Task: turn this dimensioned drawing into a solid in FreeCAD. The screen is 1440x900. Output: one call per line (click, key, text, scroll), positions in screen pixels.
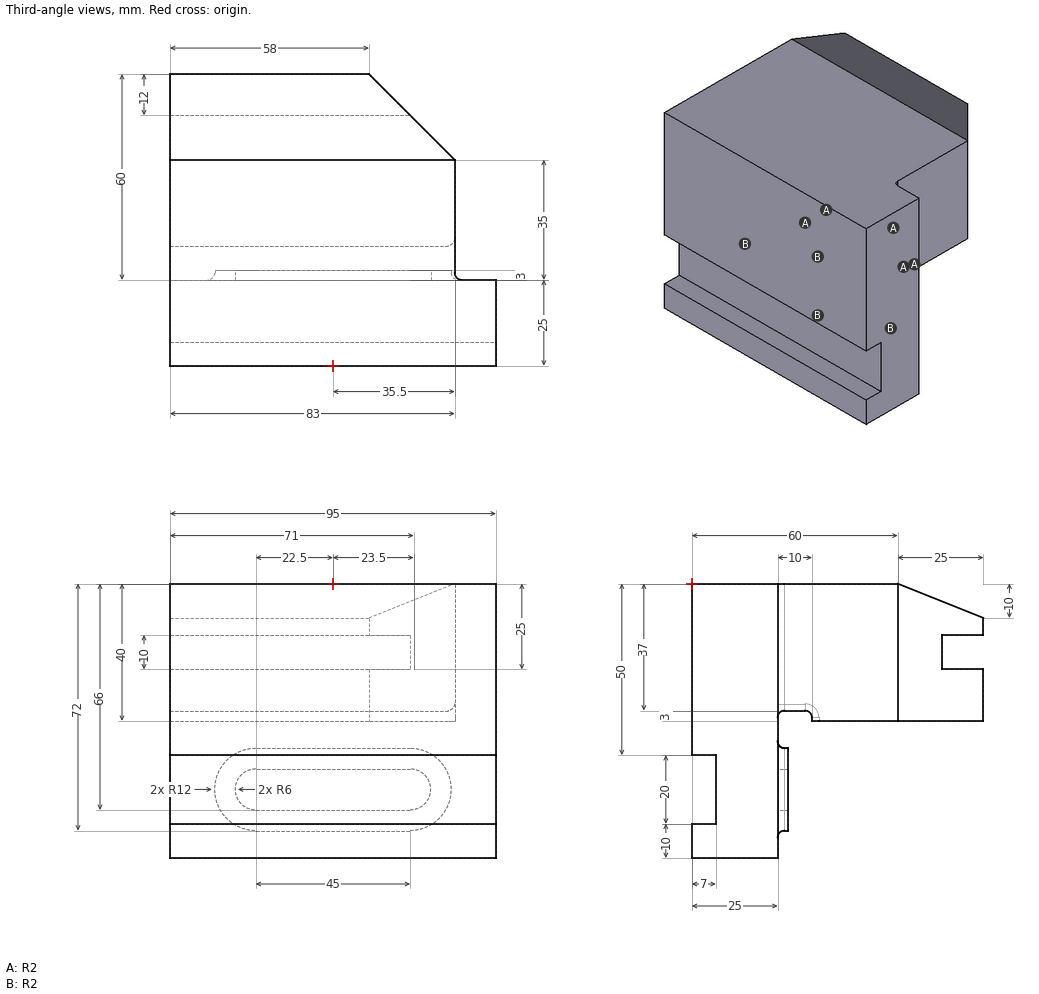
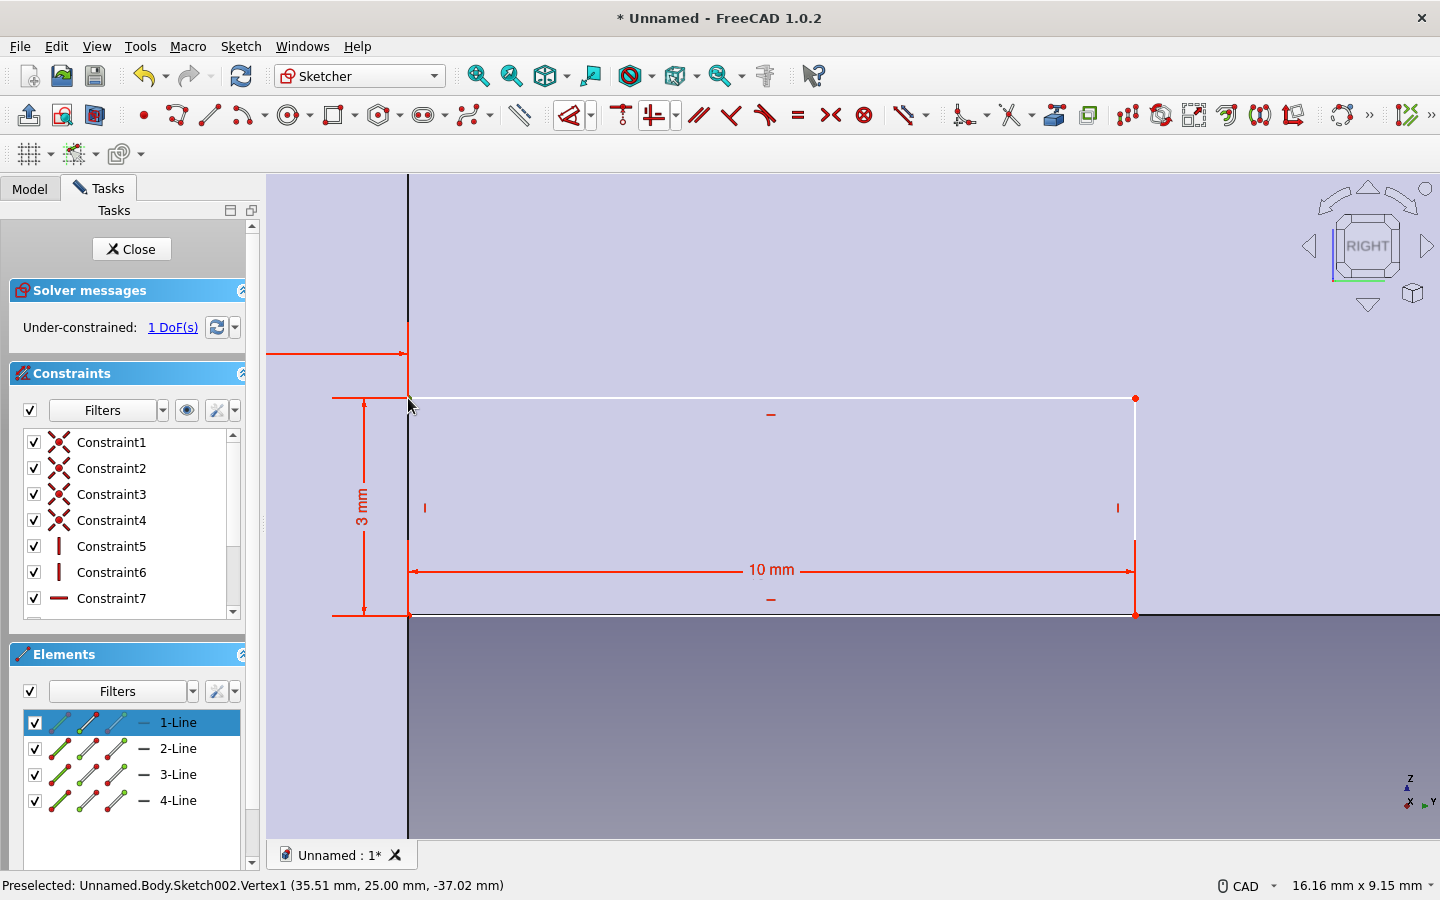
click(590, 116)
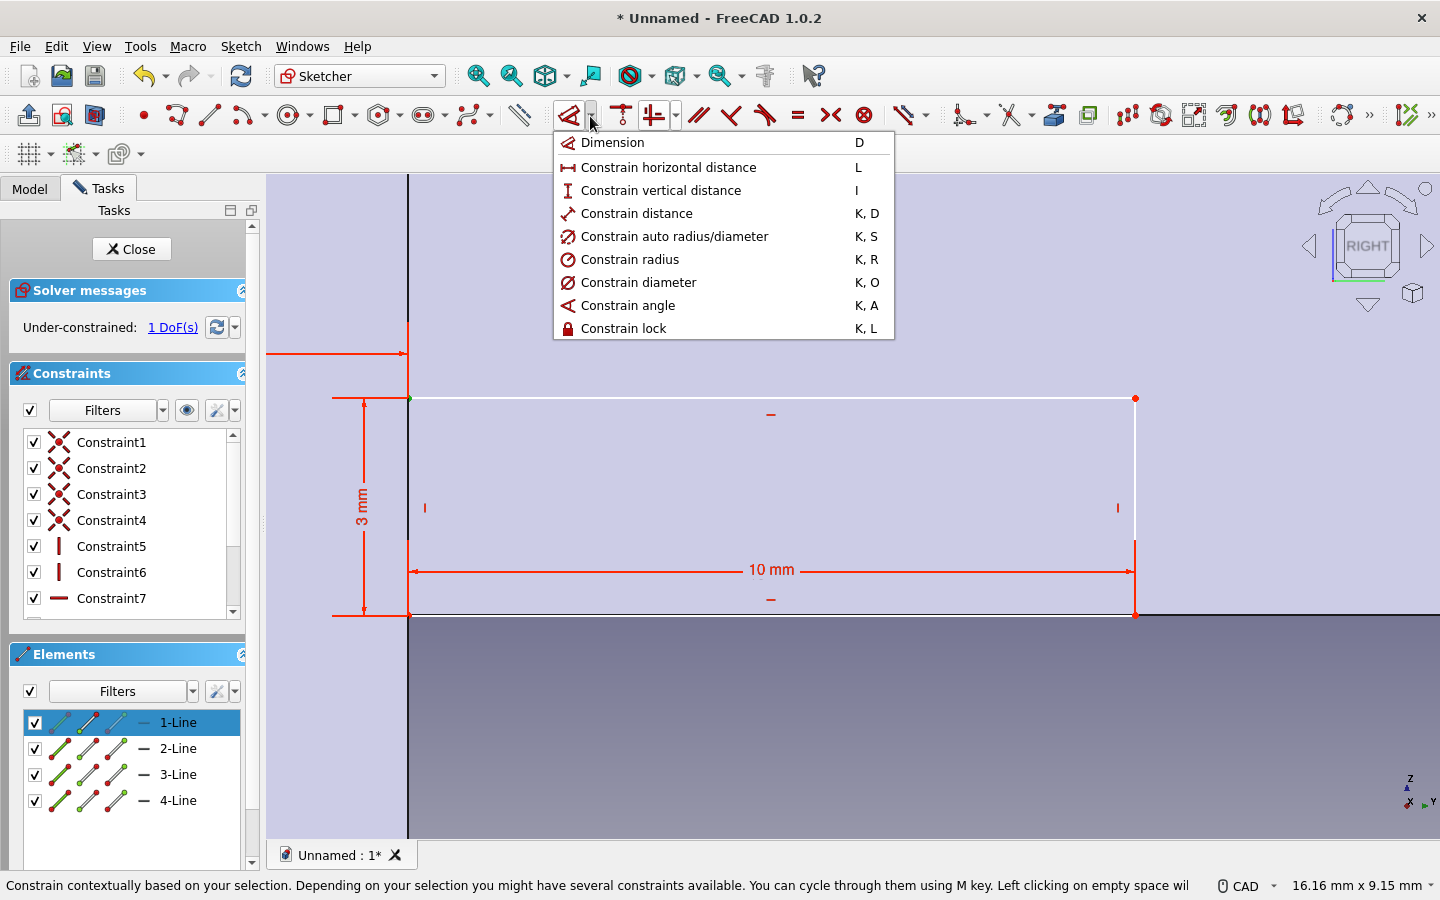
click(724, 190)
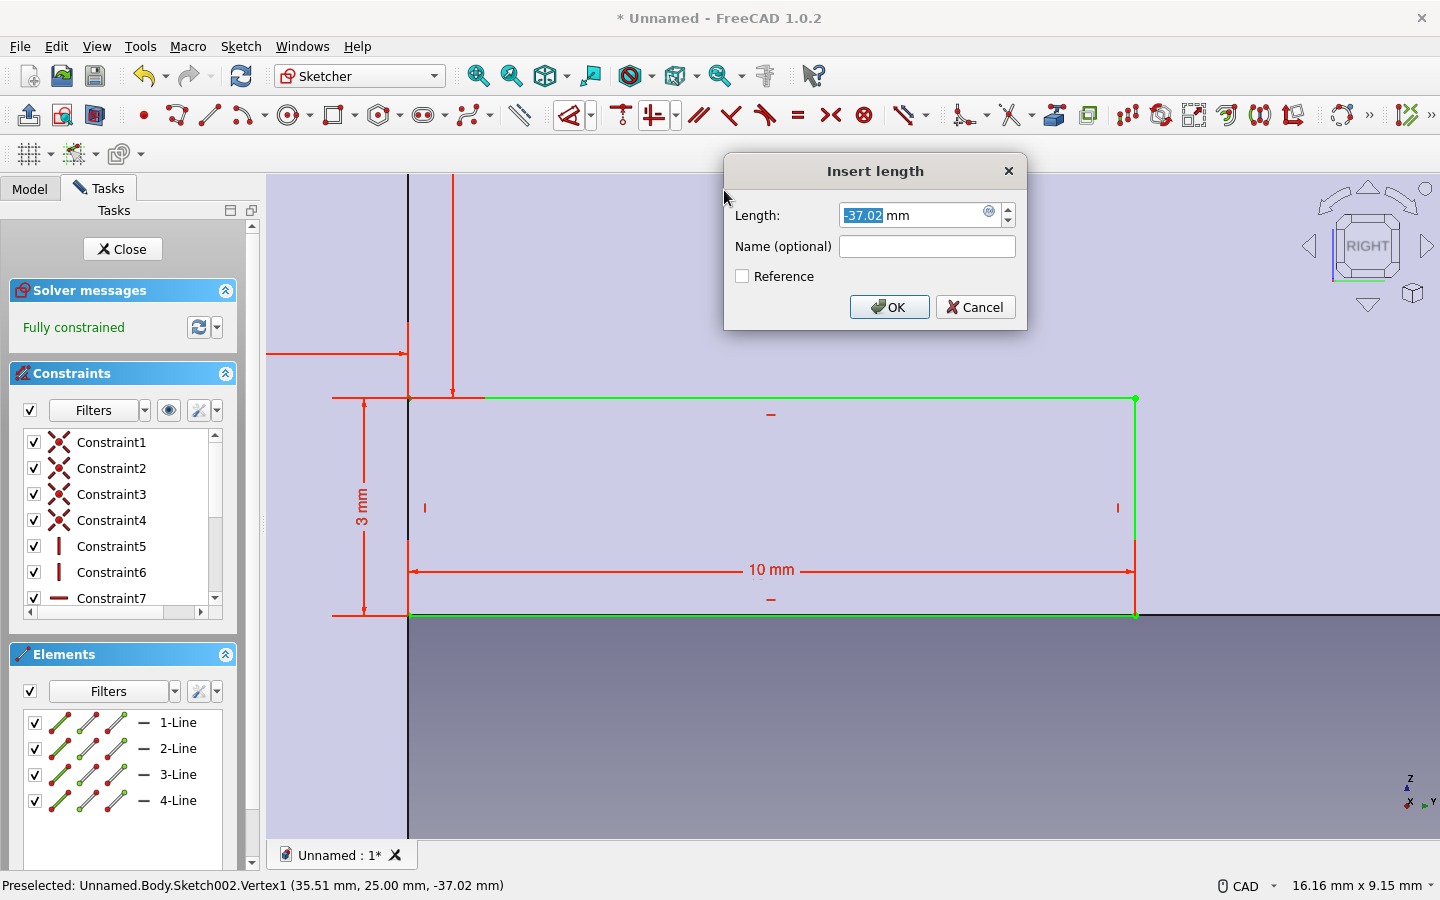
text(-37)
key(Return)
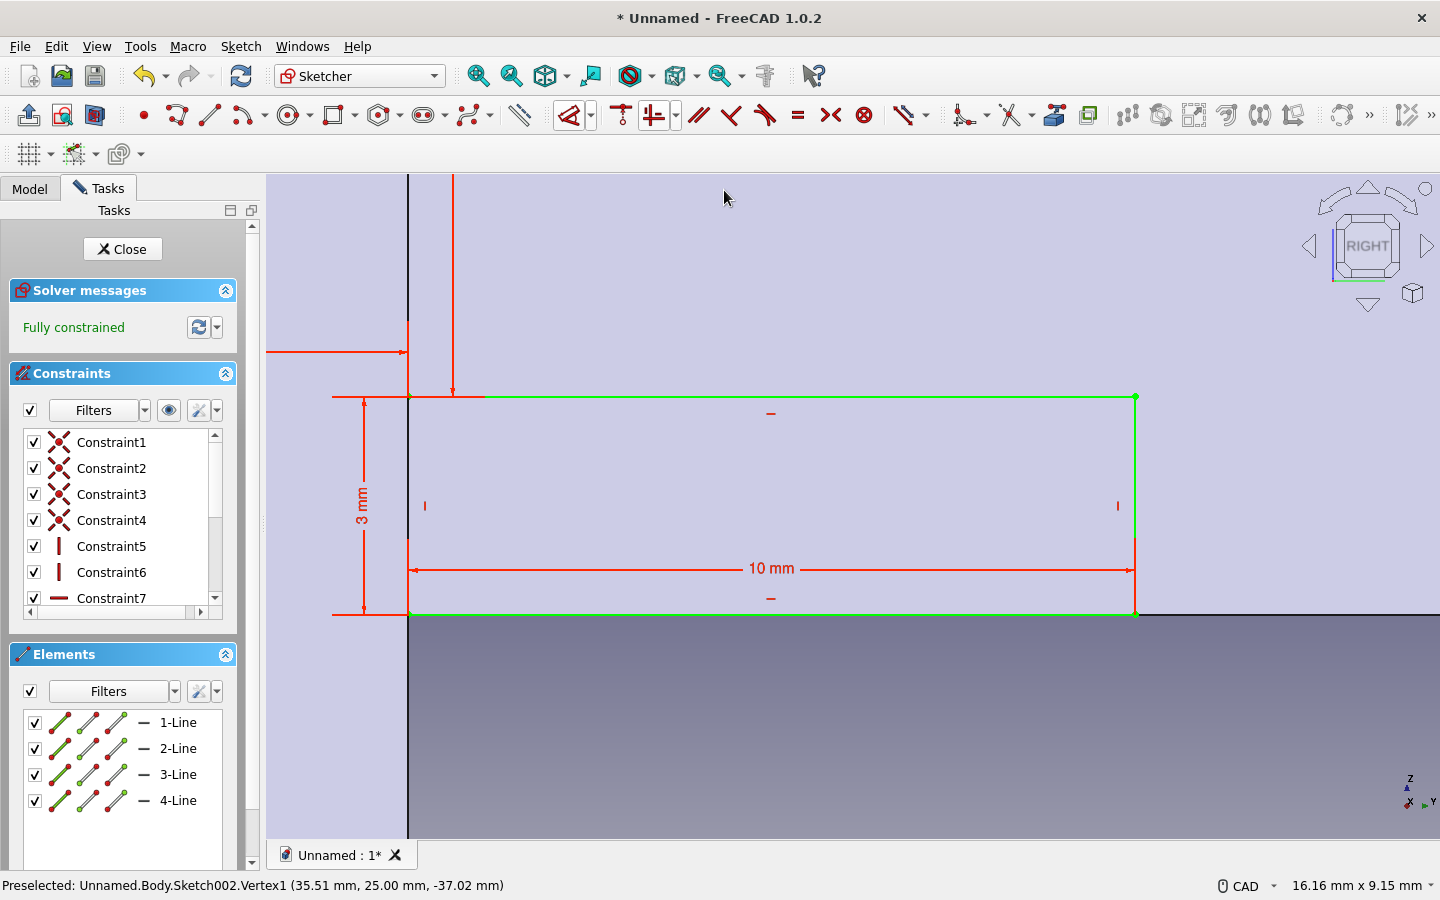
click(123, 249)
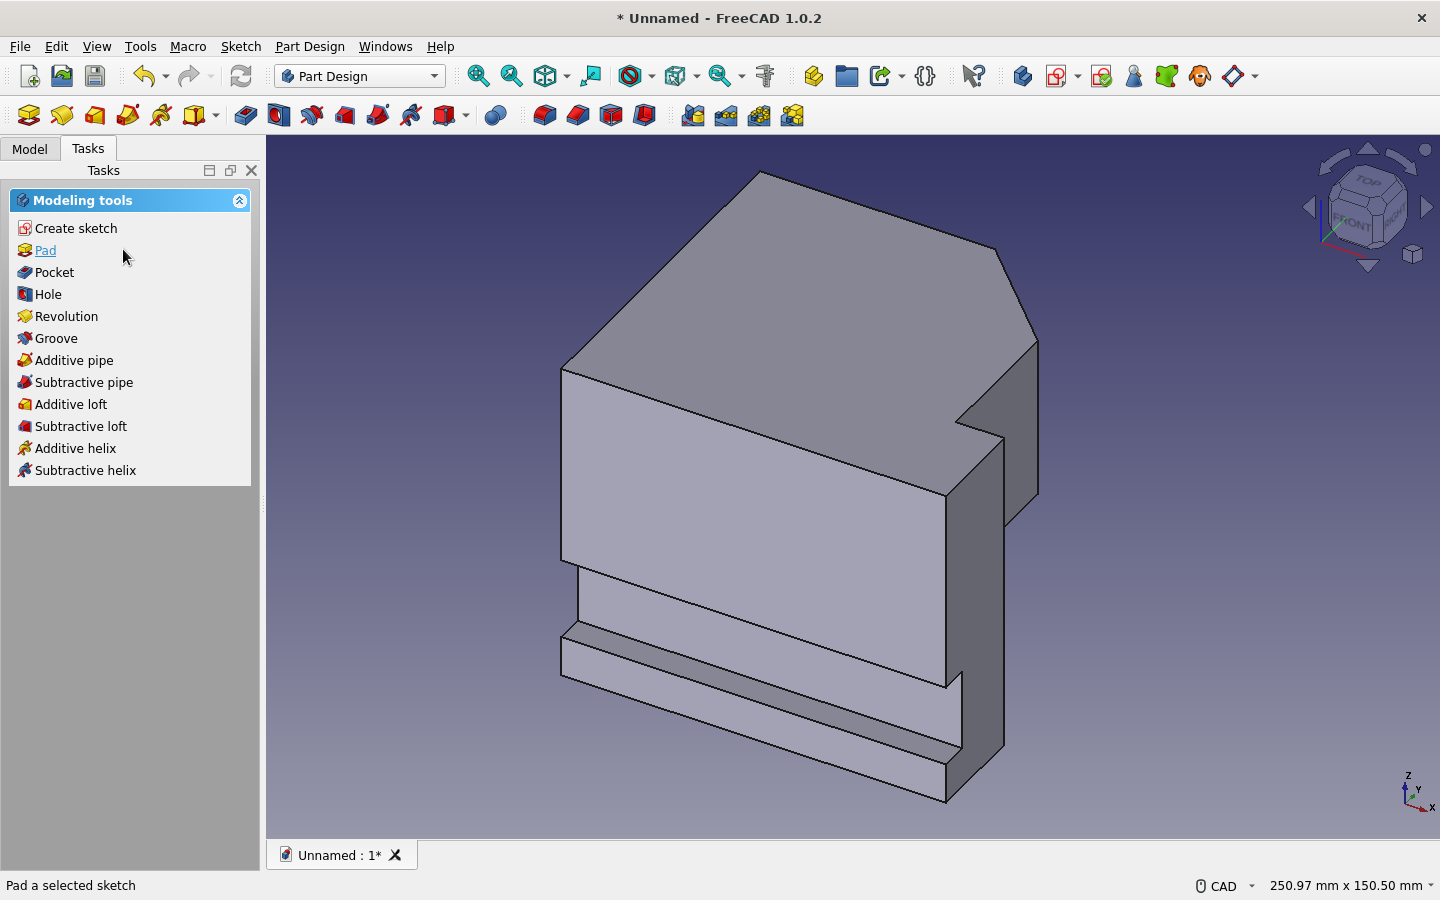
click(246, 116)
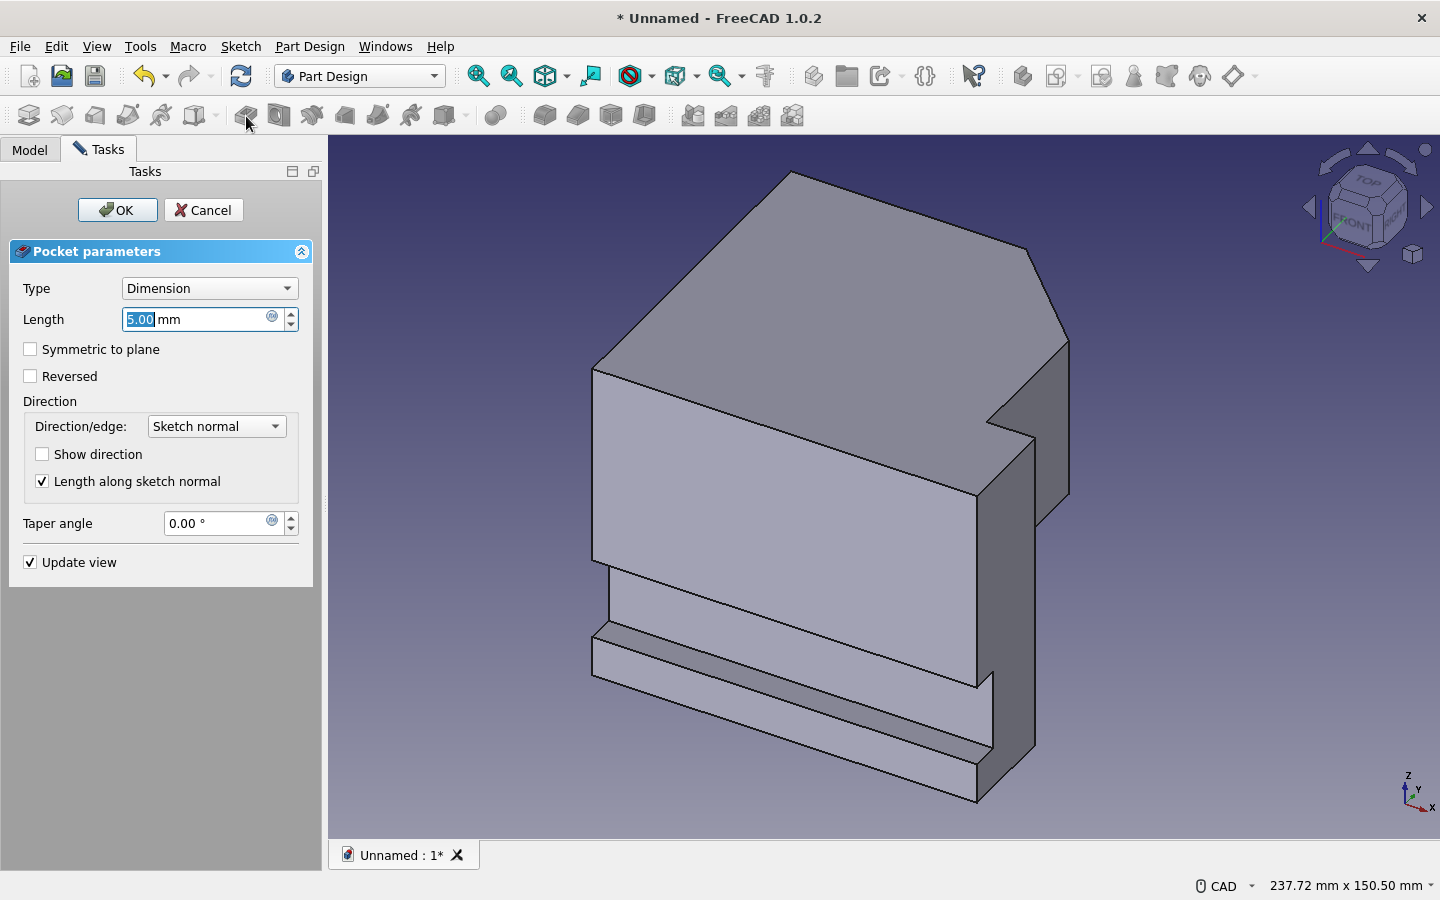
click(210, 288)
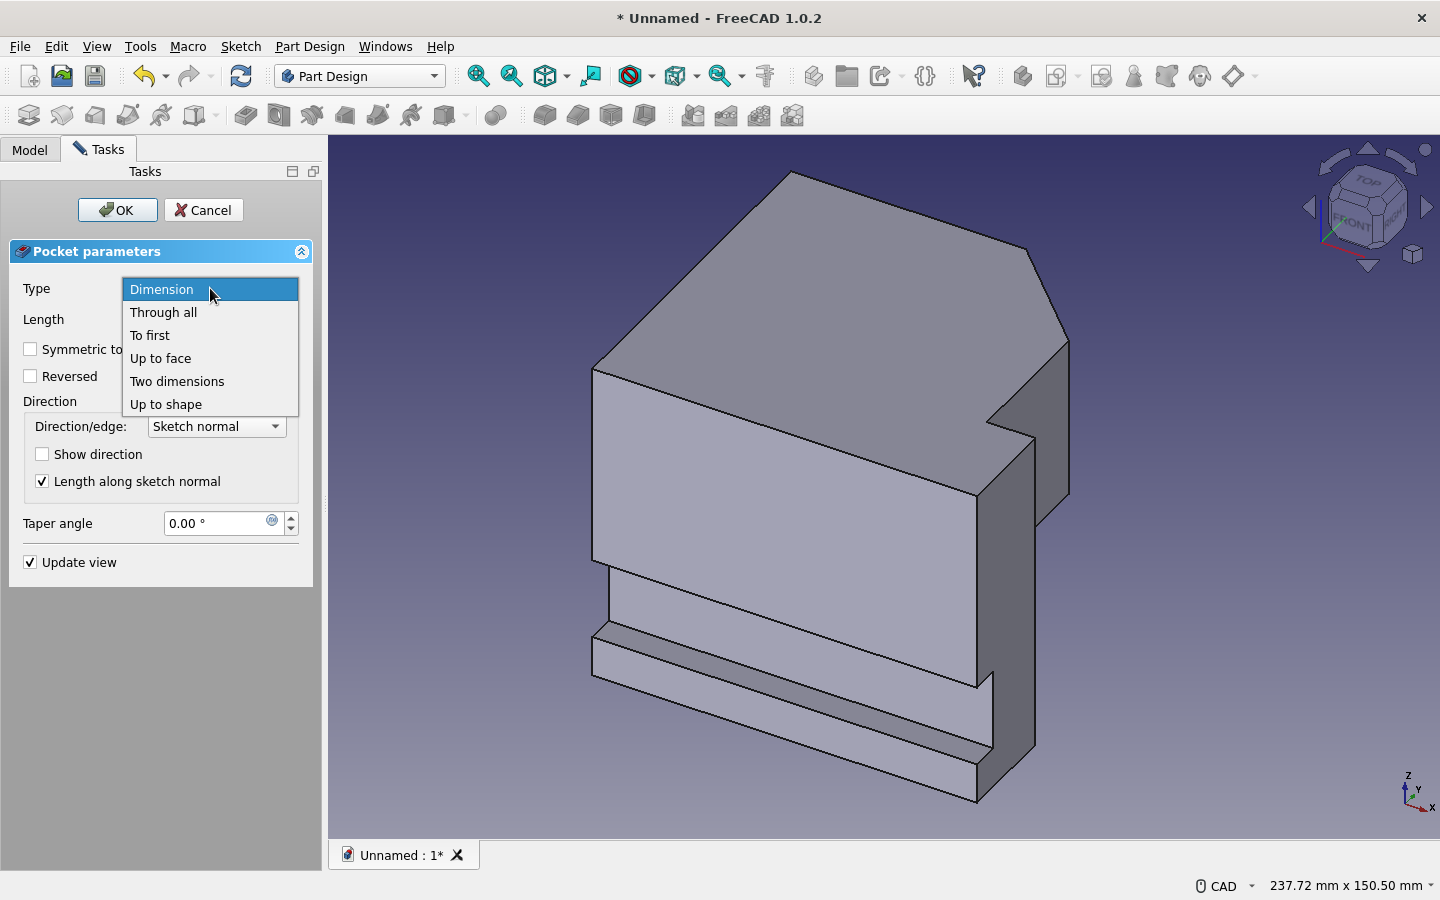
click(208, 312)